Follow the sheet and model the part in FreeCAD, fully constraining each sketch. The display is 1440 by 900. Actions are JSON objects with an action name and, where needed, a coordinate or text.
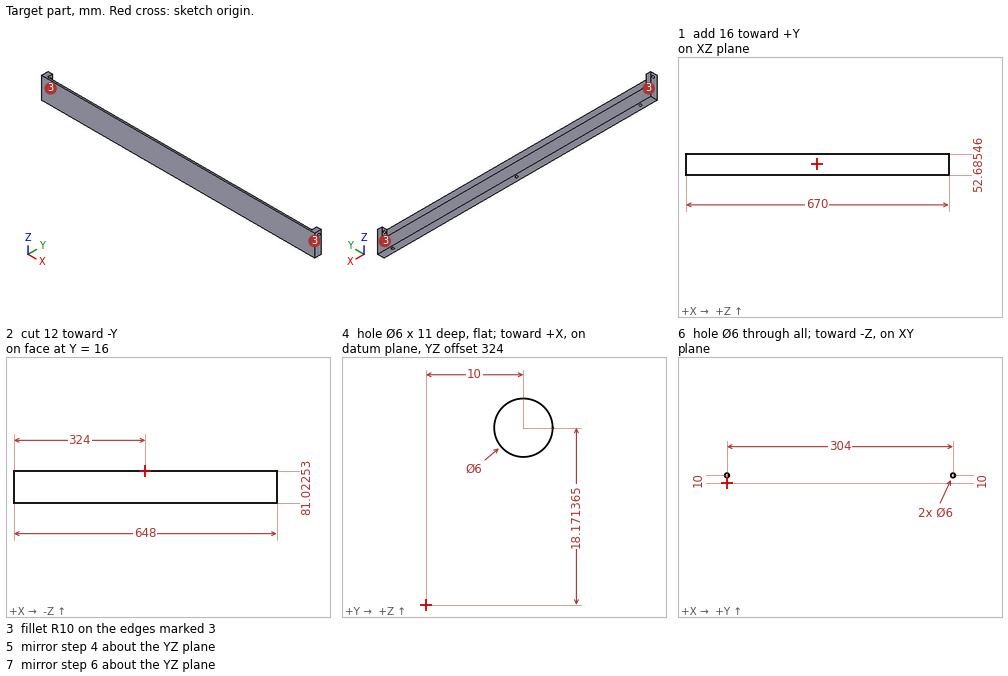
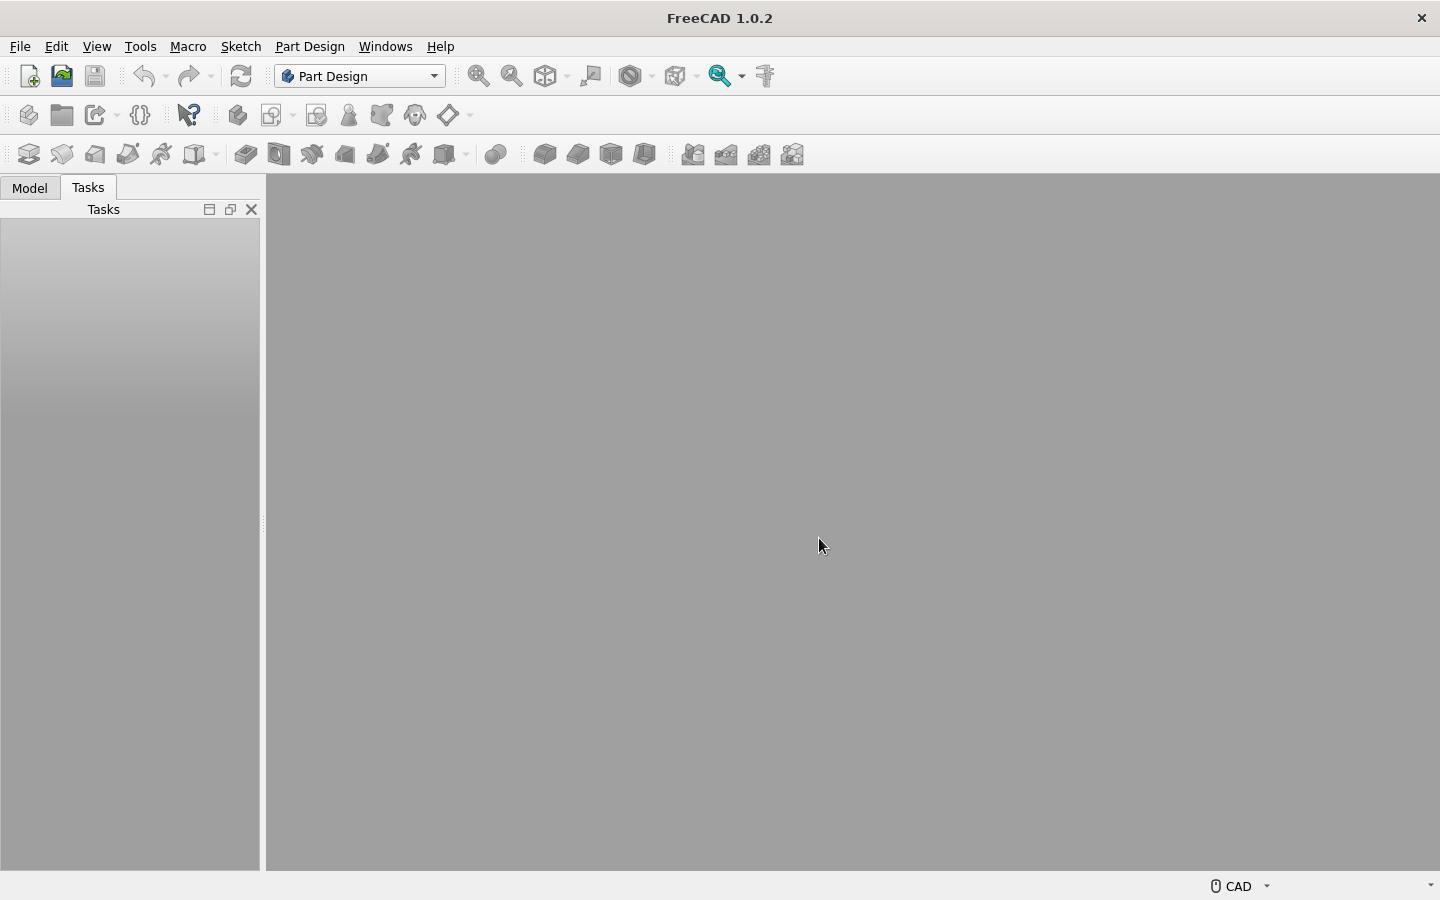
{"action": "left_click", "coordinate": [29, 76]}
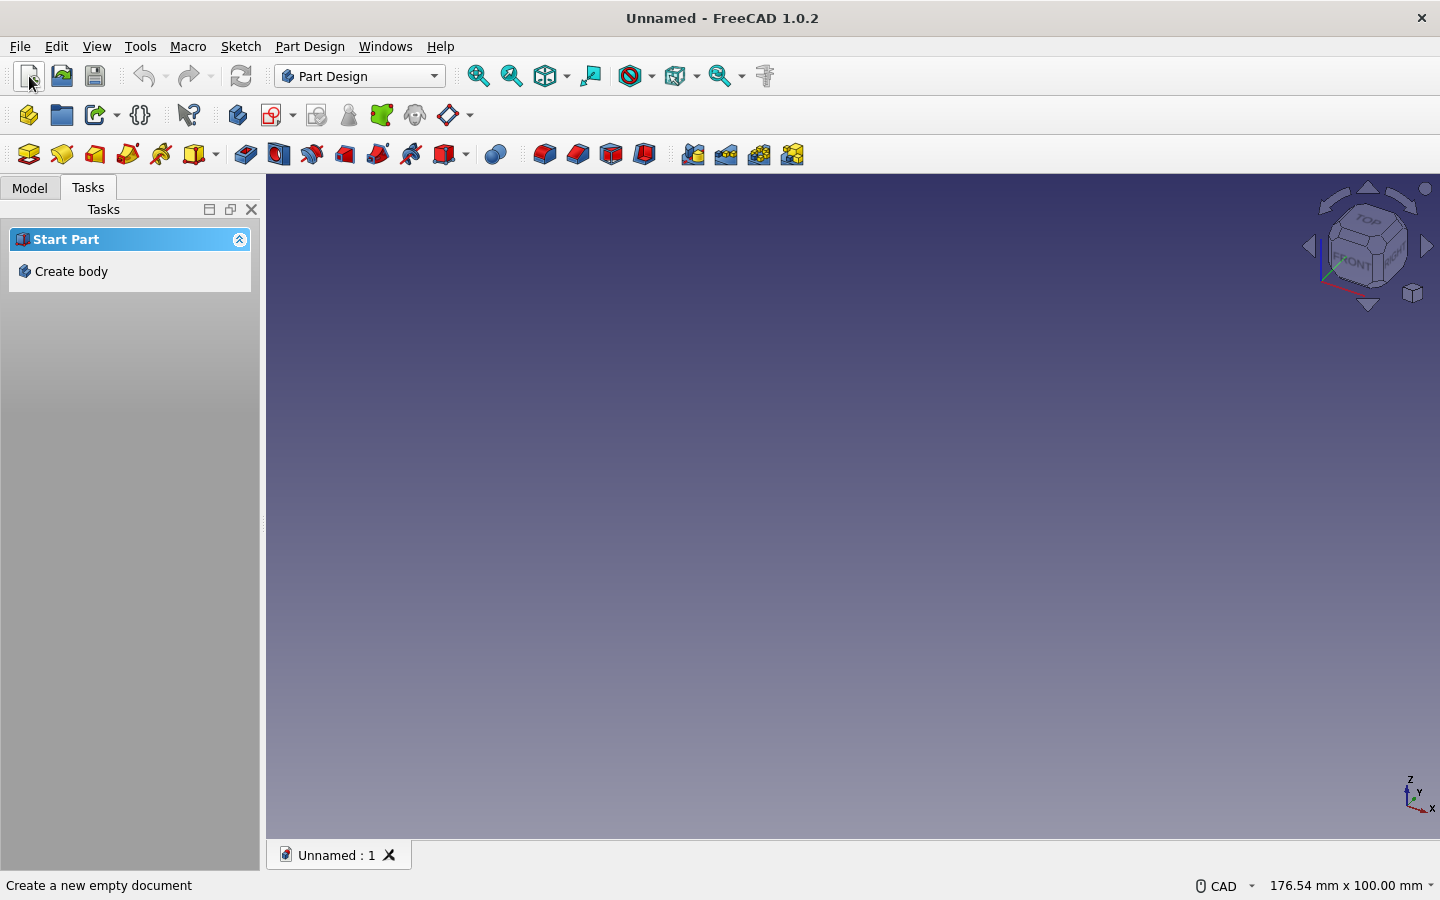
{"action": "left_click", "coordinate": [270, 116]}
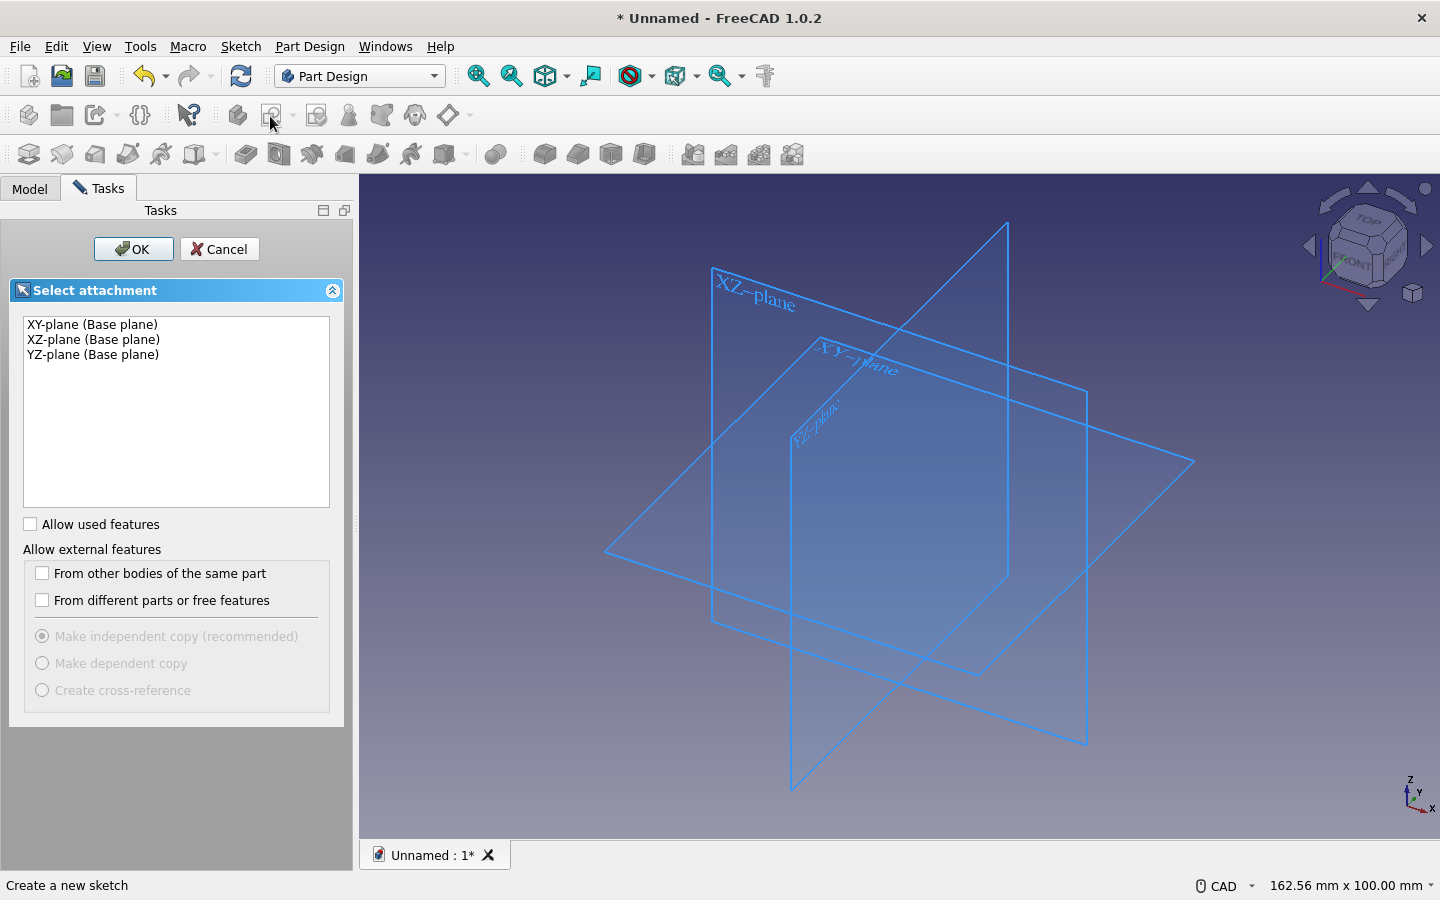
{"action": "left_click", "coordinate": [84, 340]}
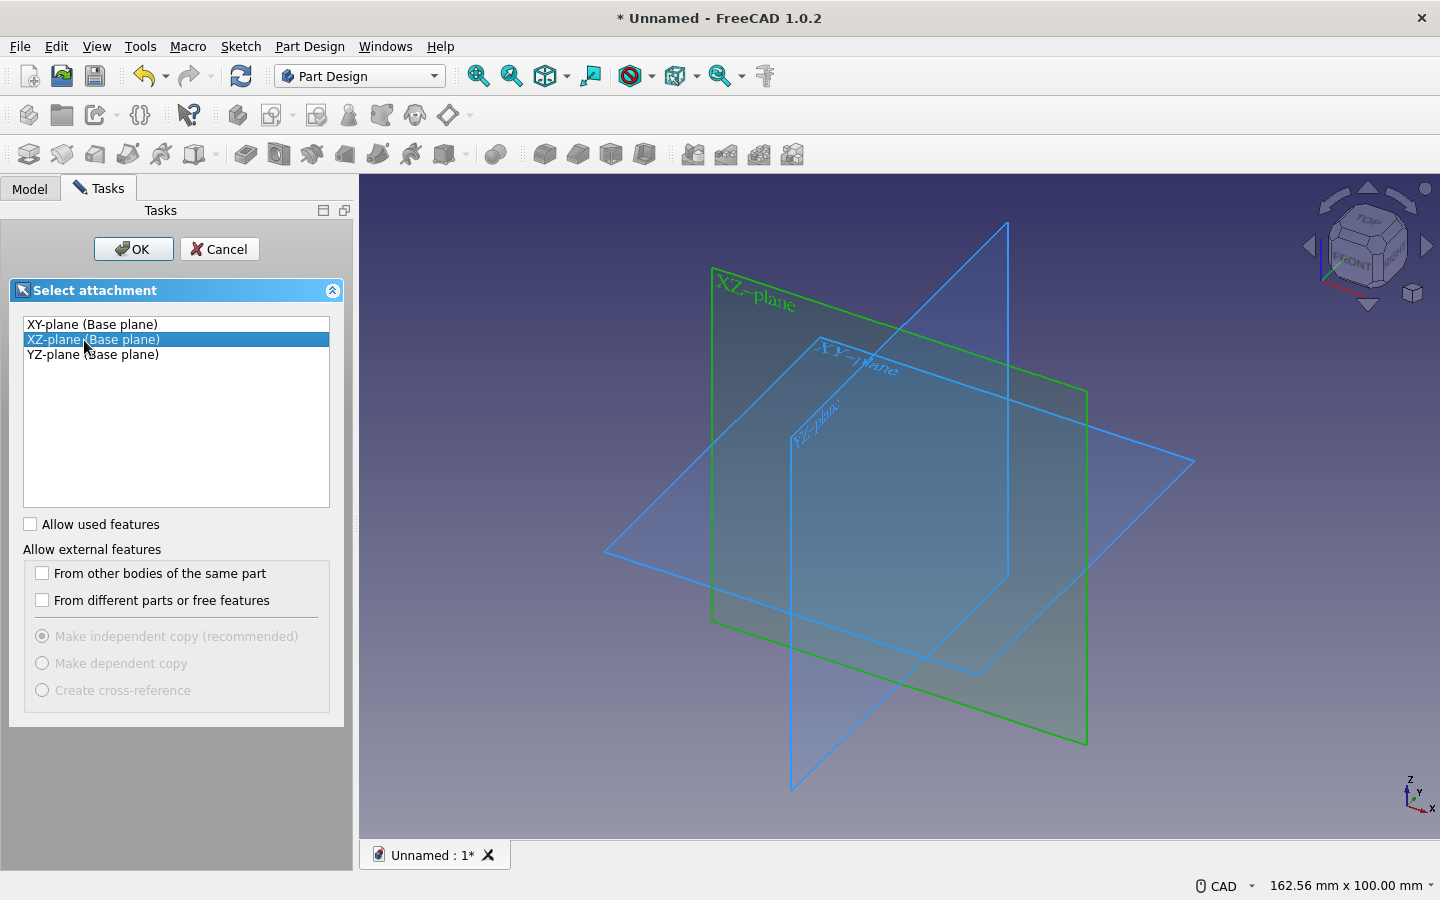
{"action": "left_click", "coordinate": [134, 249]}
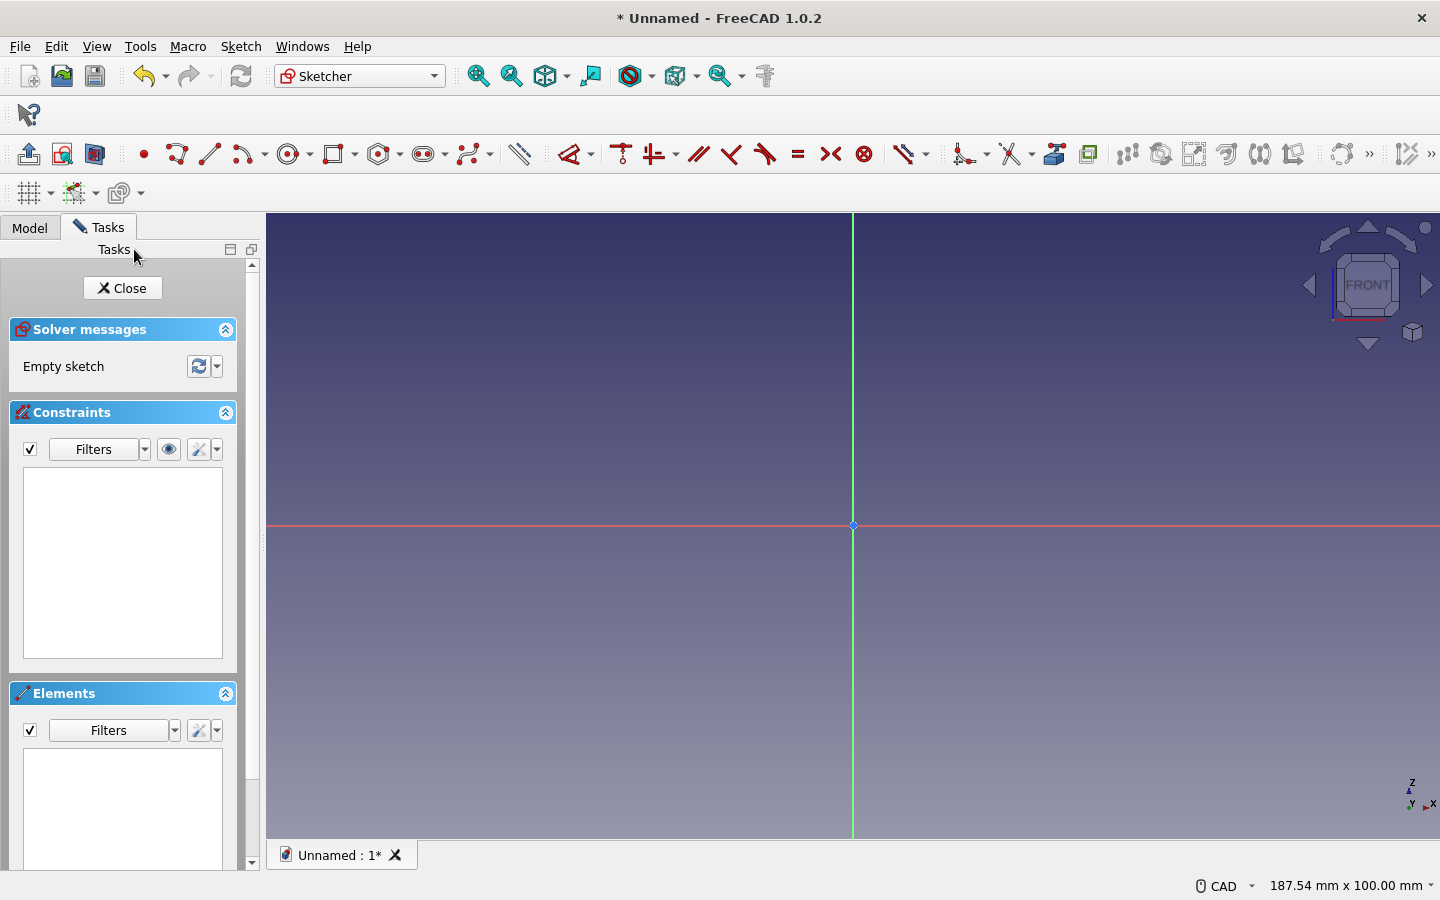
{"action": "scroll", "coordinate": [771, 526], "scroll_direction": "down", "scroll_amount": 9}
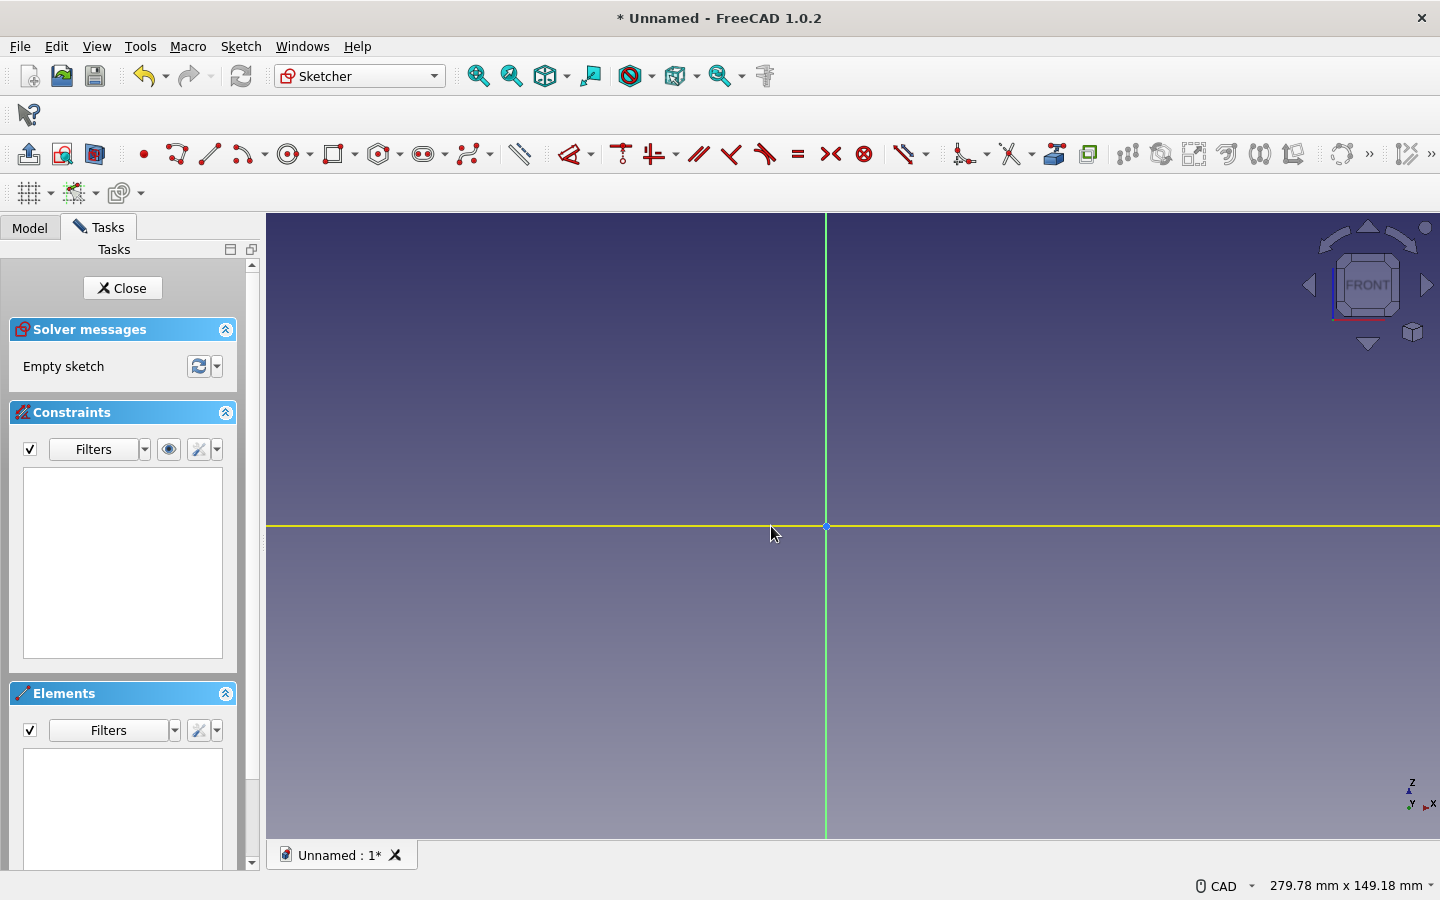
{"action": "key", "text": "g v"}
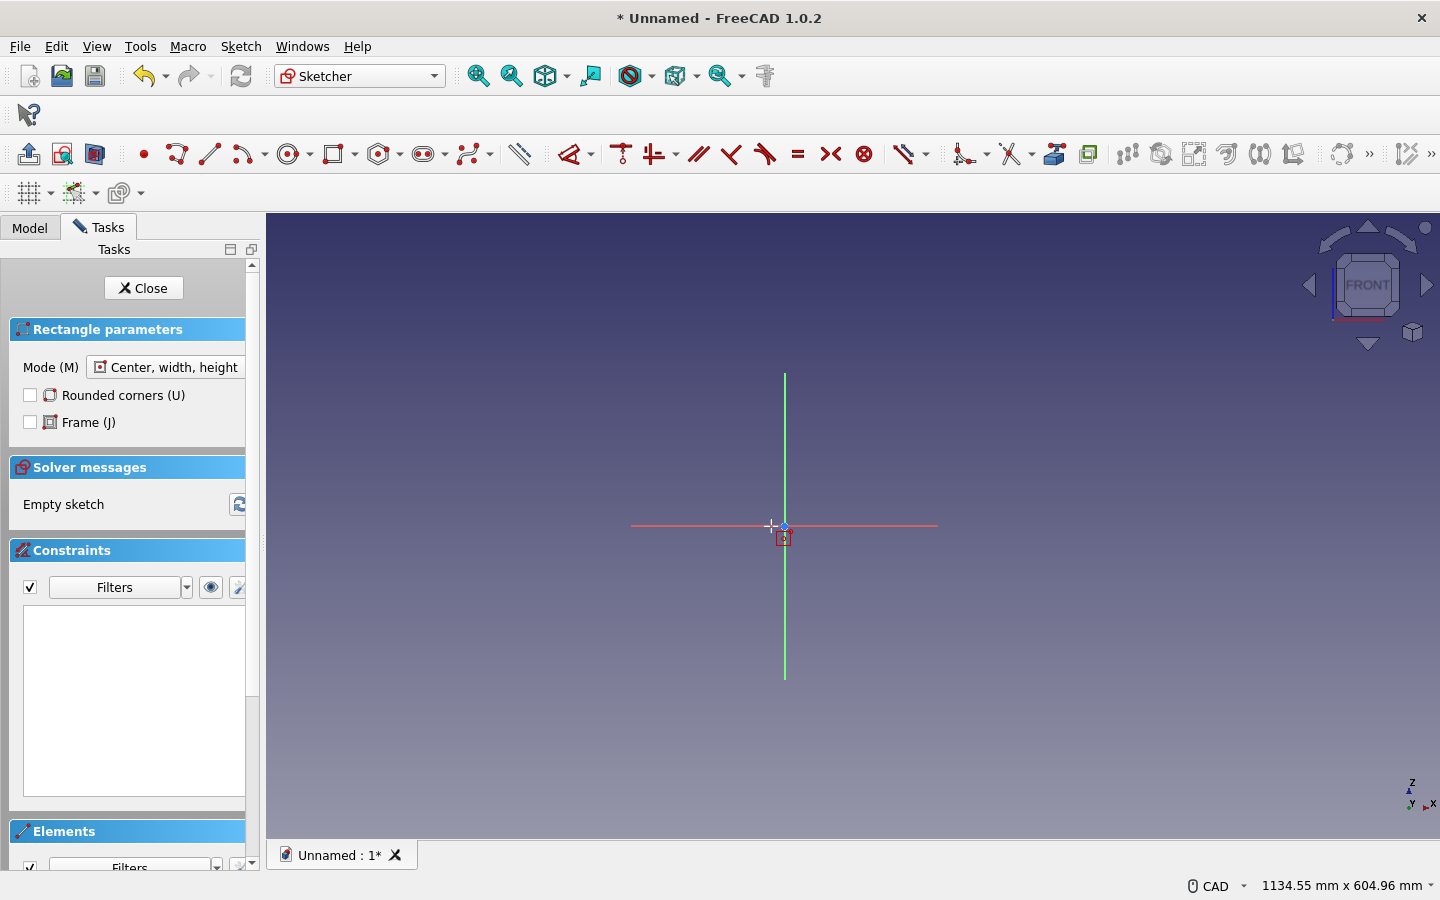
{"action": "left_click", "coordinate": [785, 526]}
{"action": "mouse_move", "coordinate": [1132, 499]}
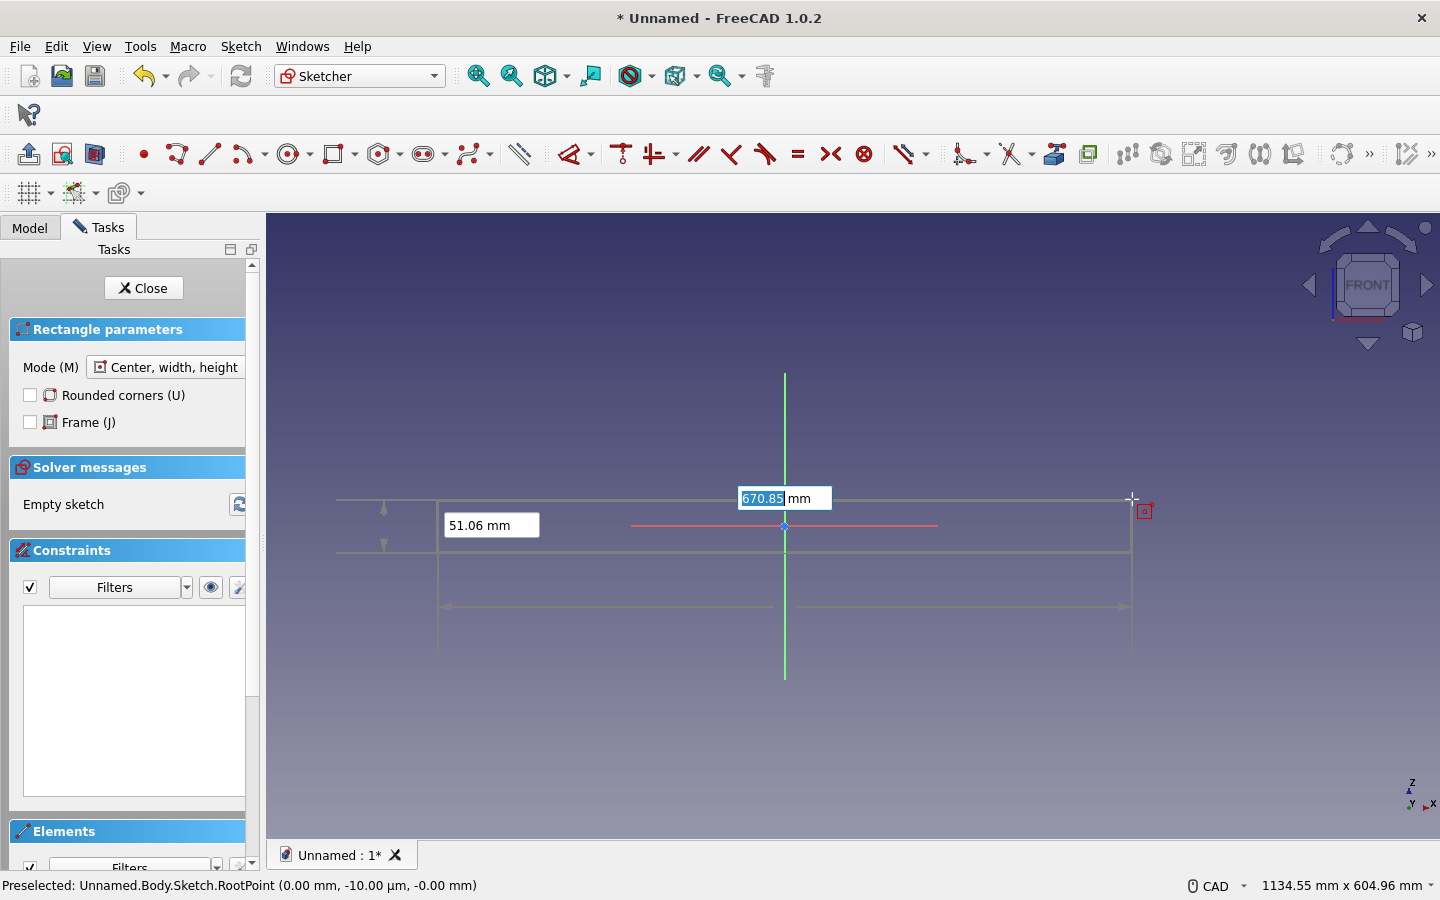
{"action": "type", "text": "670"}
{"action": "key", "text": "Tab"}
{"action": "type", "text": "52.68546"}
{"action": "key", "text": "Return"}
{"action": "key", "text": "Escape"}